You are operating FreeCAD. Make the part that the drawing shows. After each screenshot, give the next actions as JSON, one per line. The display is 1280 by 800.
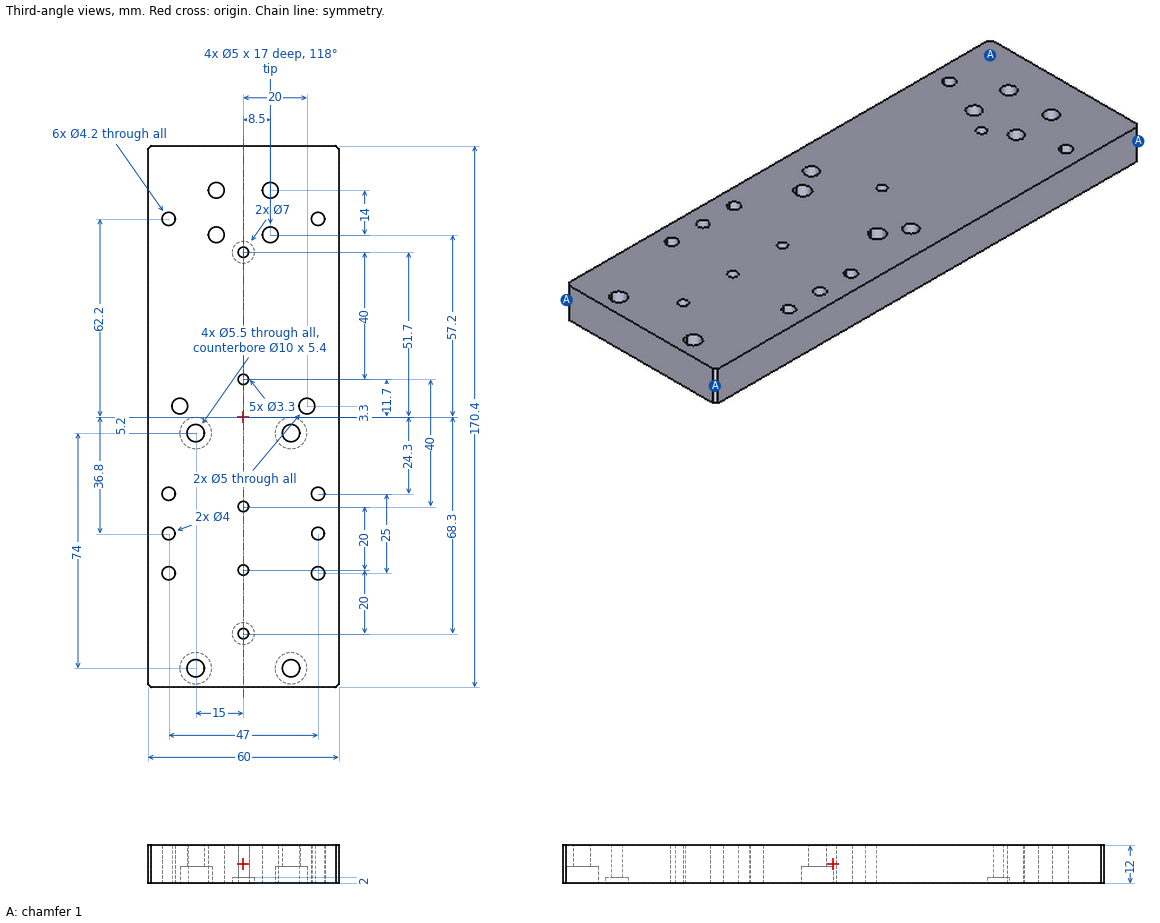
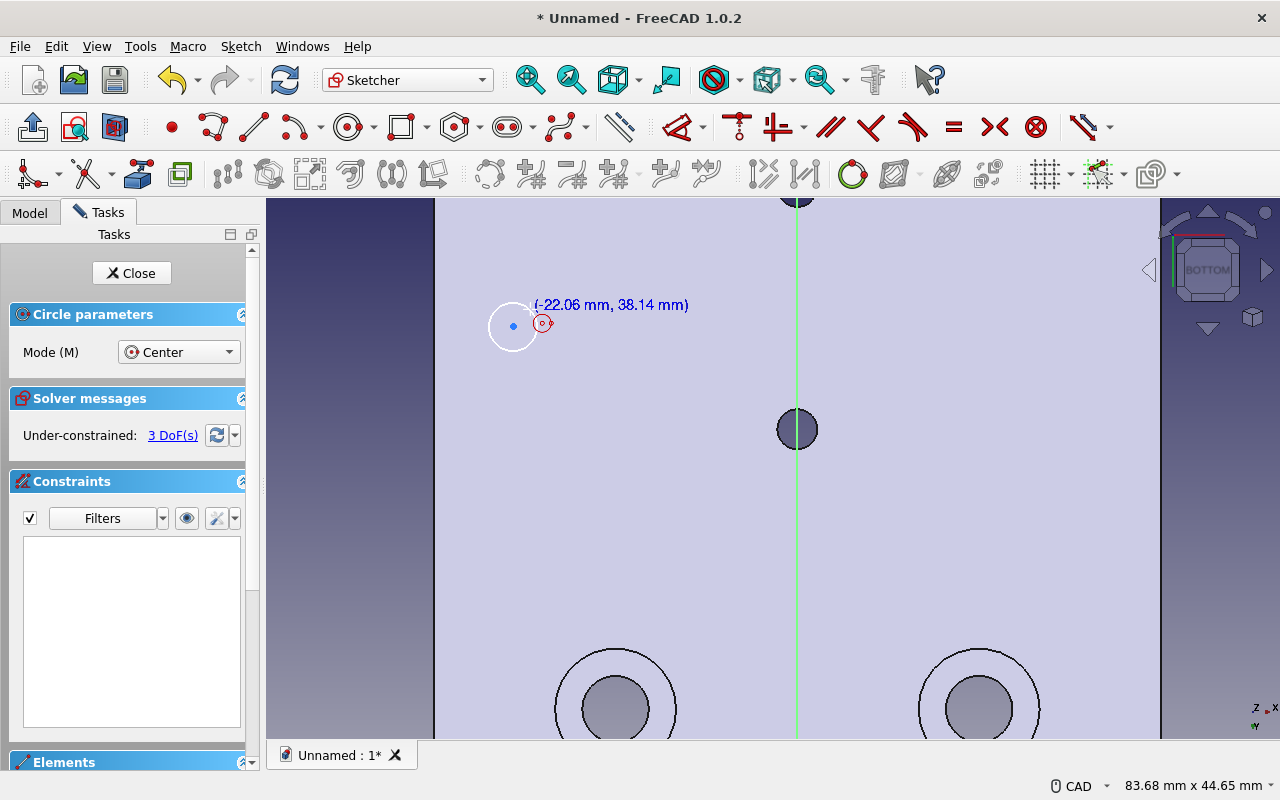
{"action": "left_click", "coordinate": [1082, 326]}
{"action": "left_click", "coordinate": [1099, 309]}
{"action": "key", "text": "Escape"}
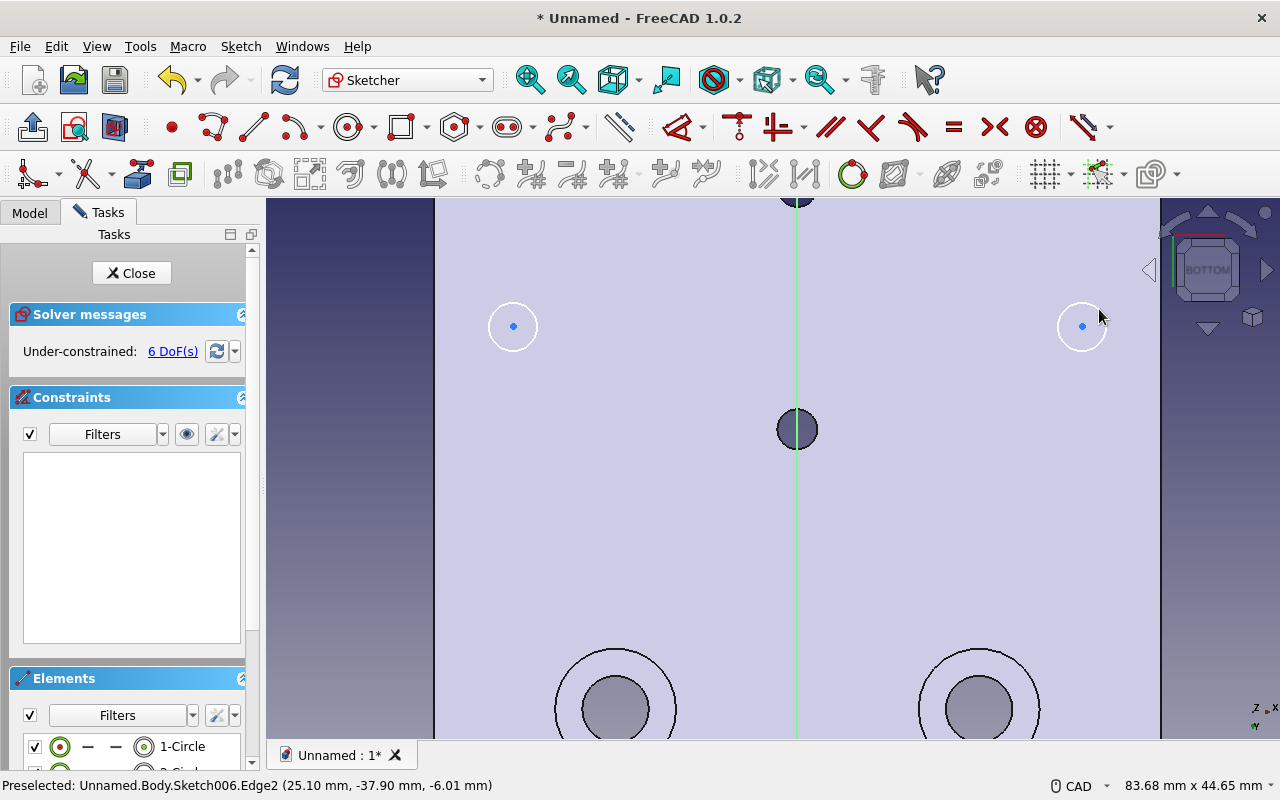
{"action": "left_click", "coordinate": [530, 310]}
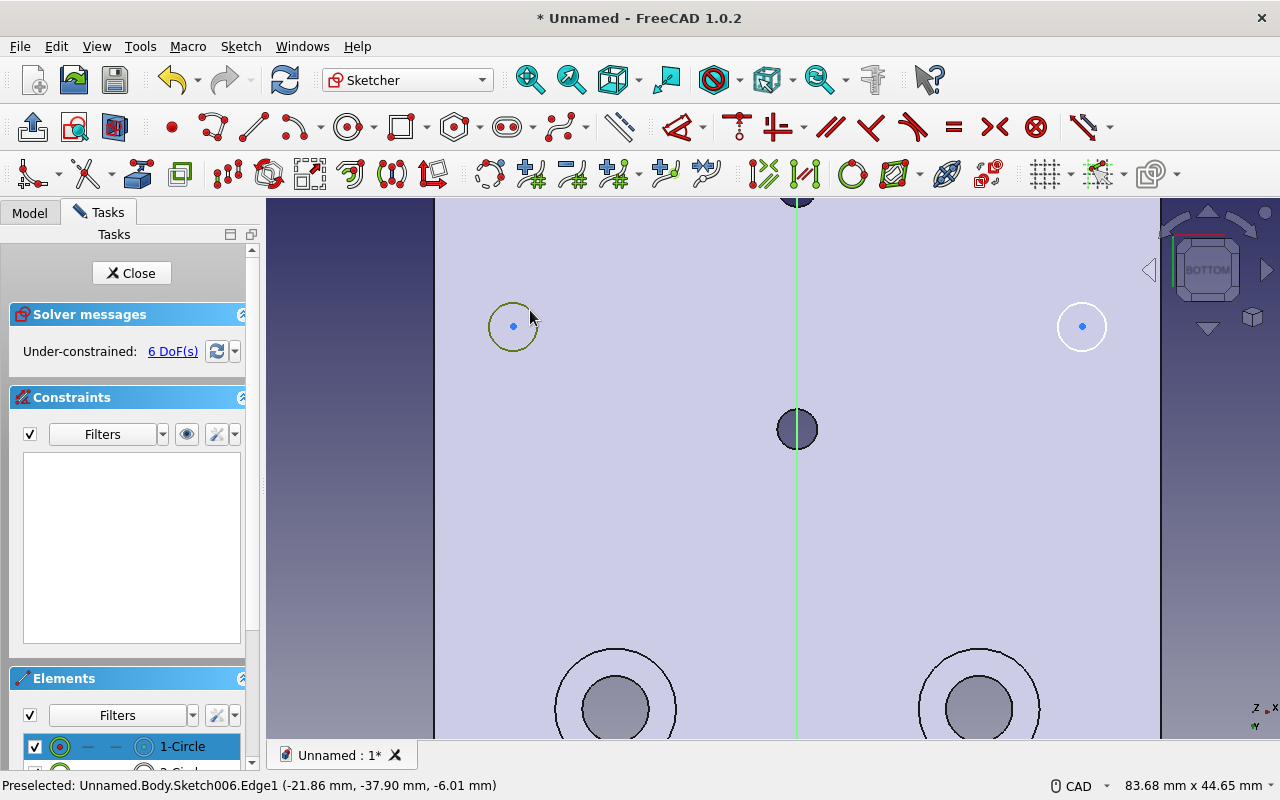
{"action": "left_click", "coordinate": [1099, 310]}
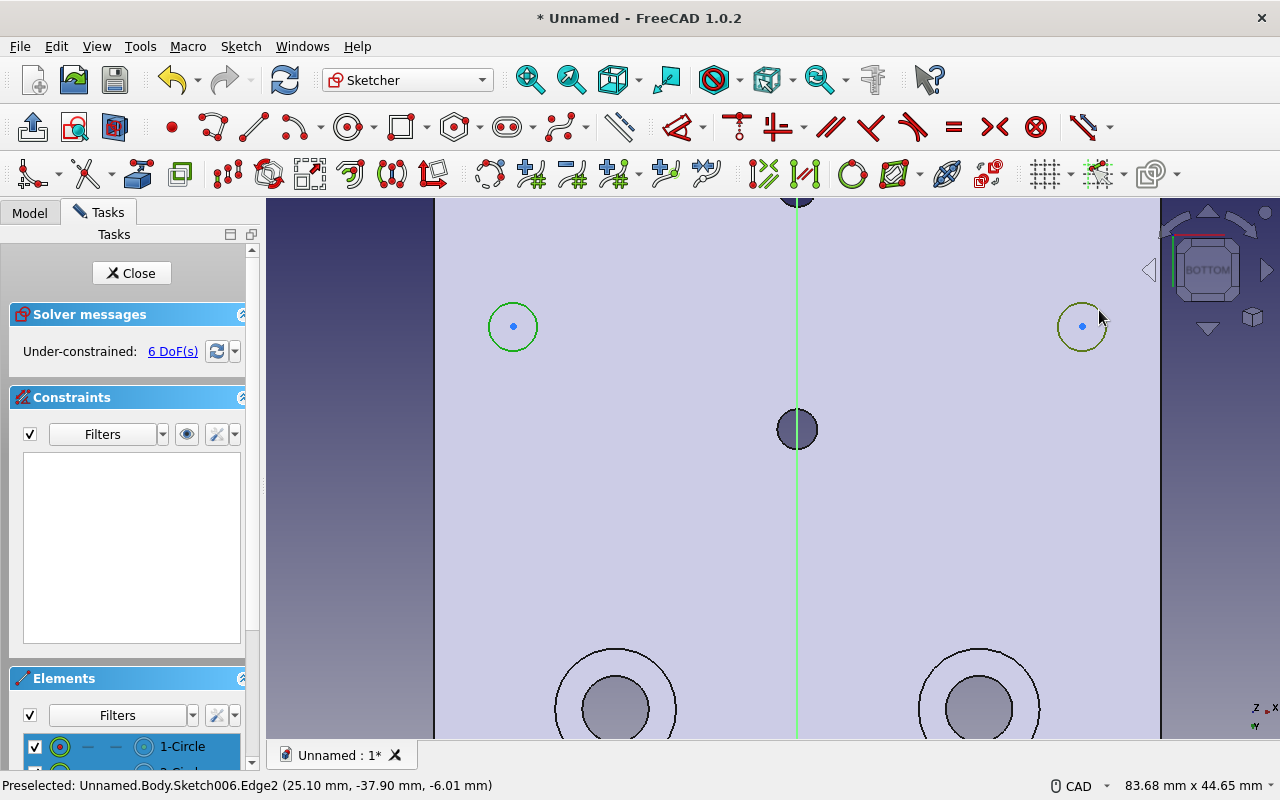
{"action": "left_click", "coordinate": [954, 128]}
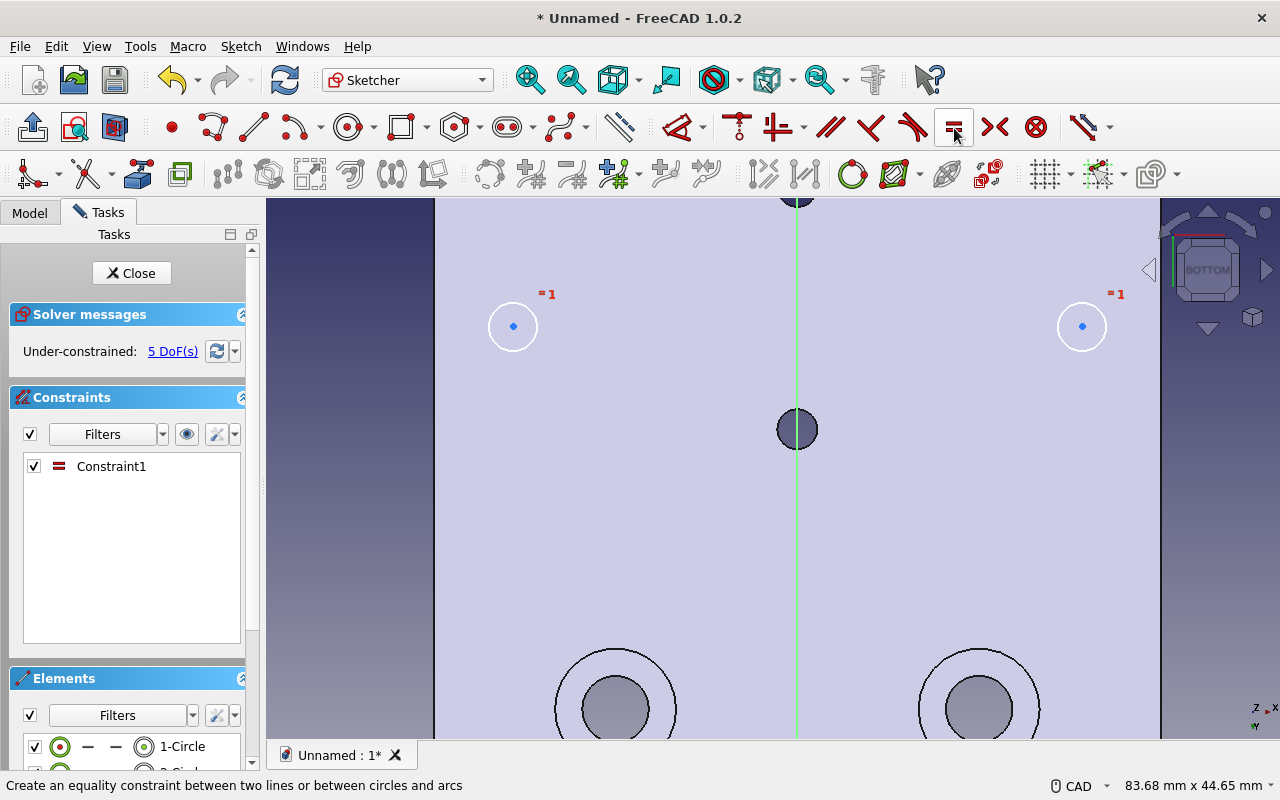
{"action": "left_click", "coordinate": [513, 327]}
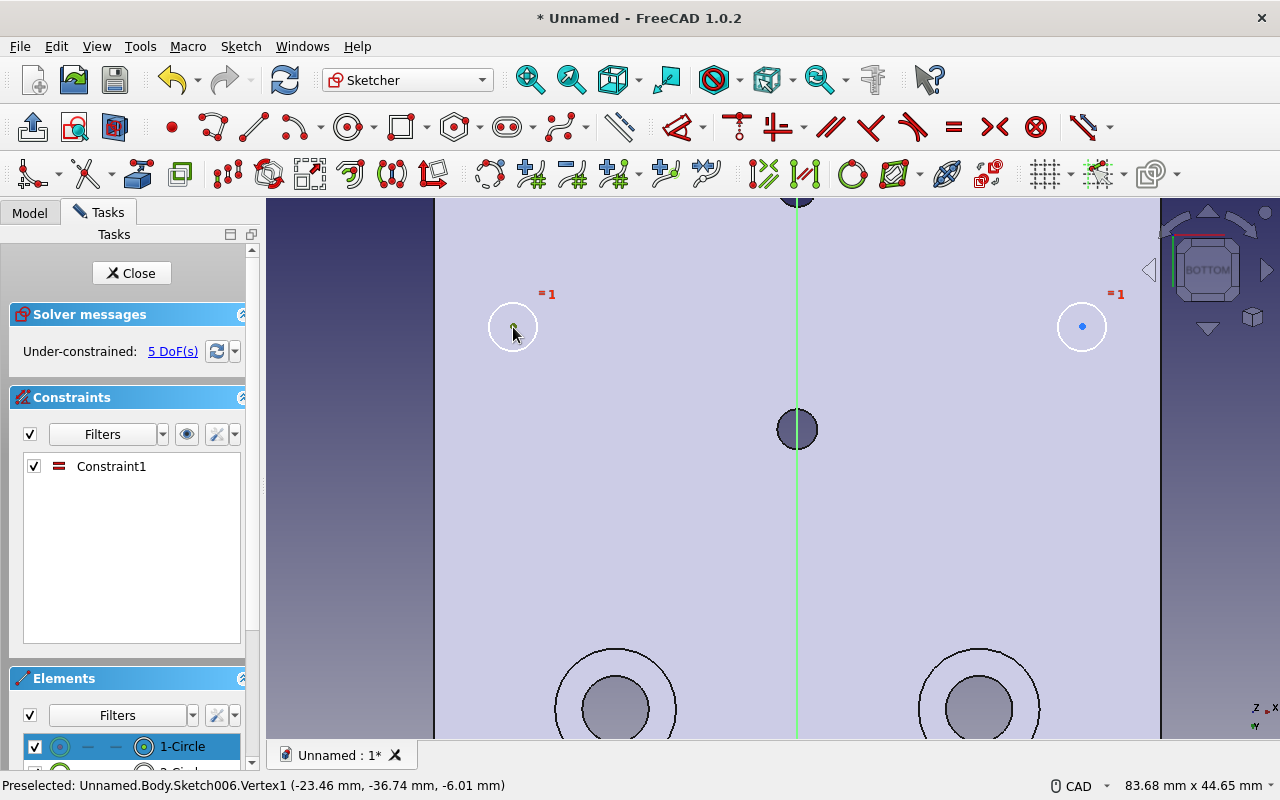
{"action": "left_click", "coordinate": [1082, 327]}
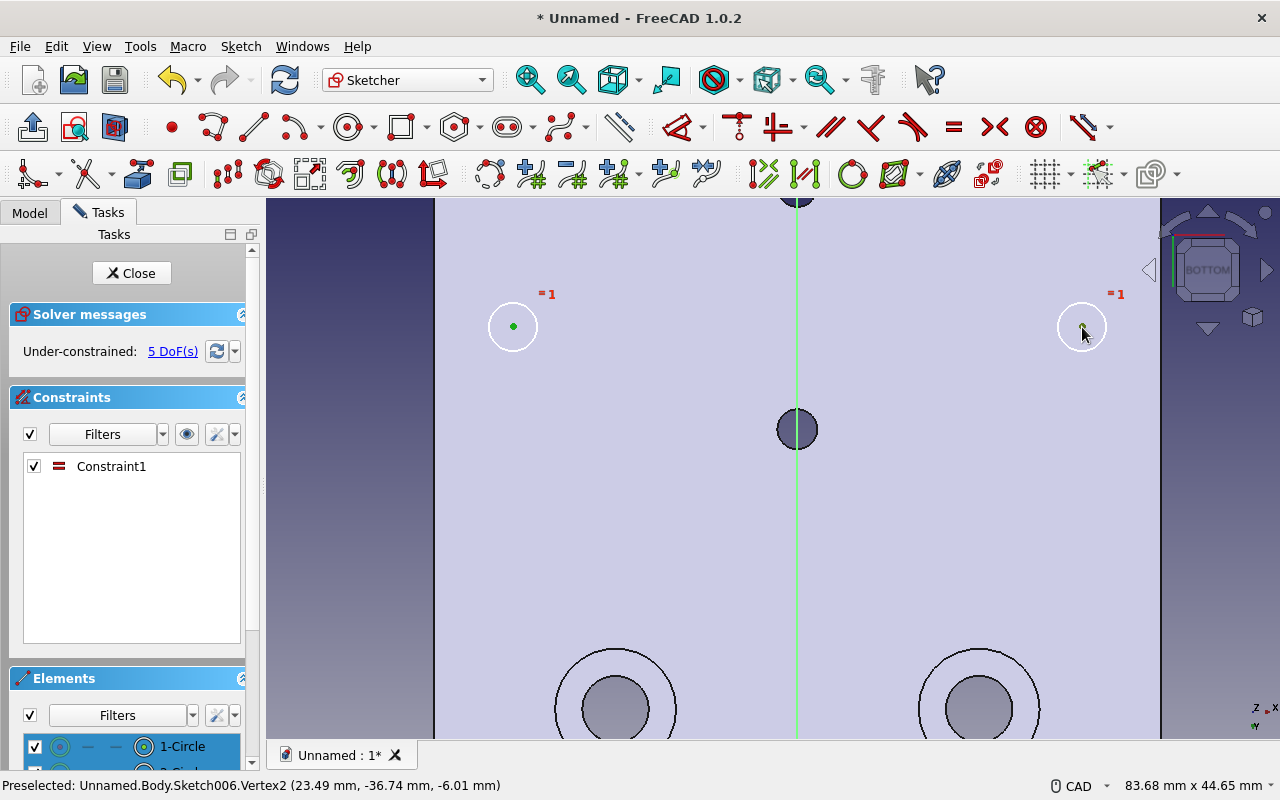
{"action": "left_click", "coordinate": [797, 676]}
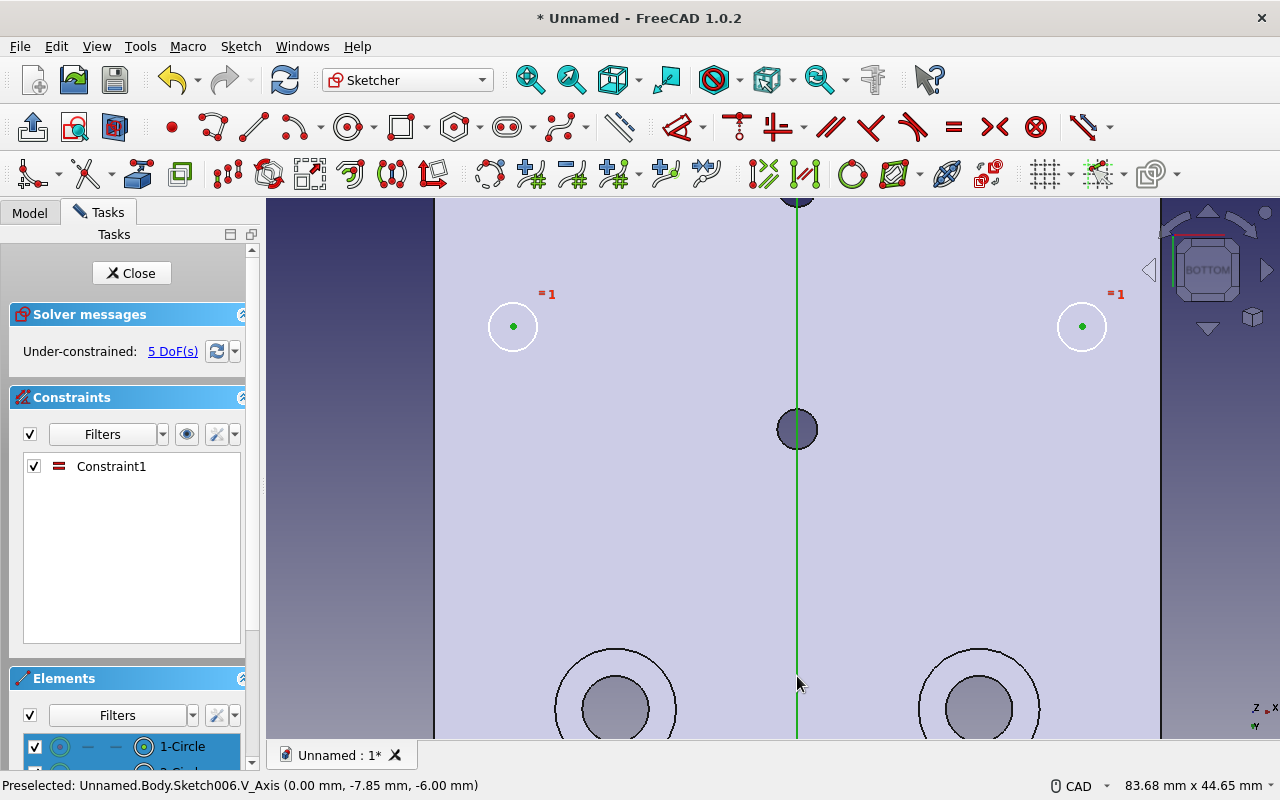
{"action": "left_click", "coordinate": [995, 128]}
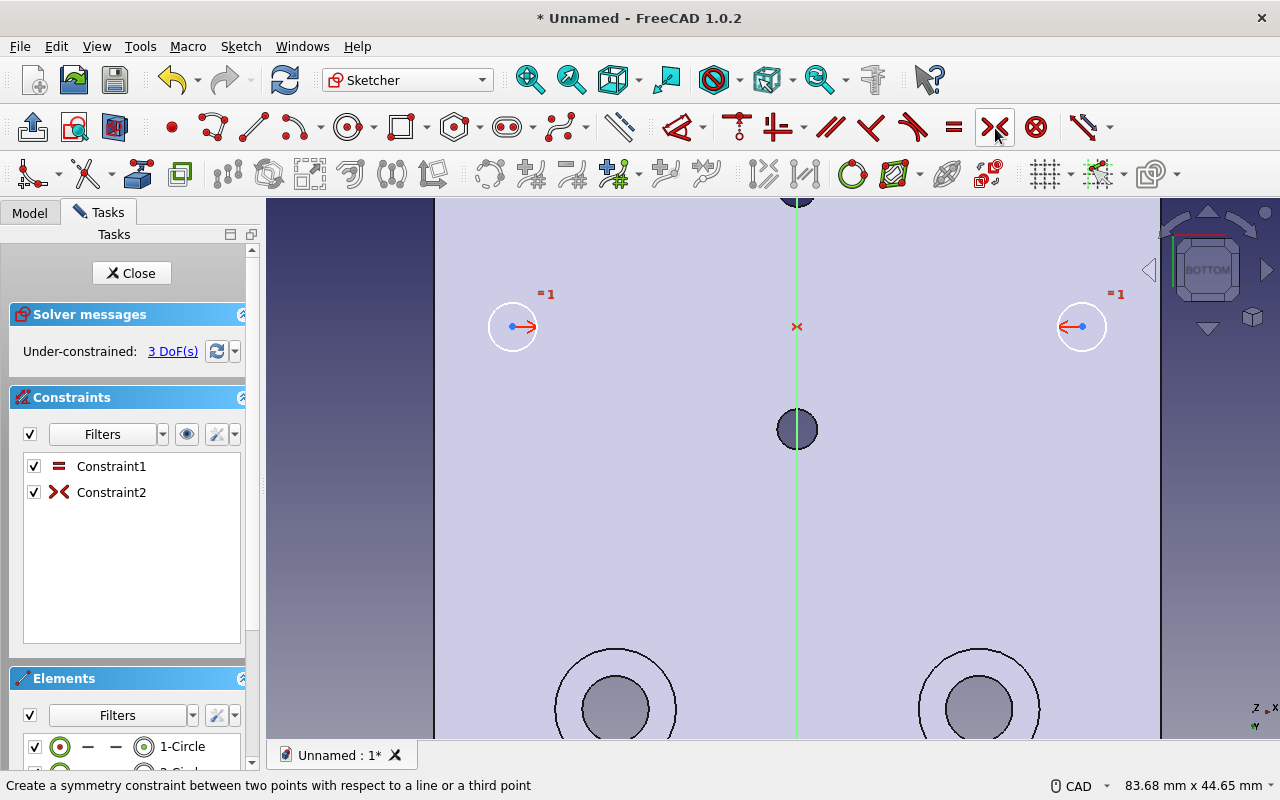
{"action": "left_click", "coordinate": [676, 128]}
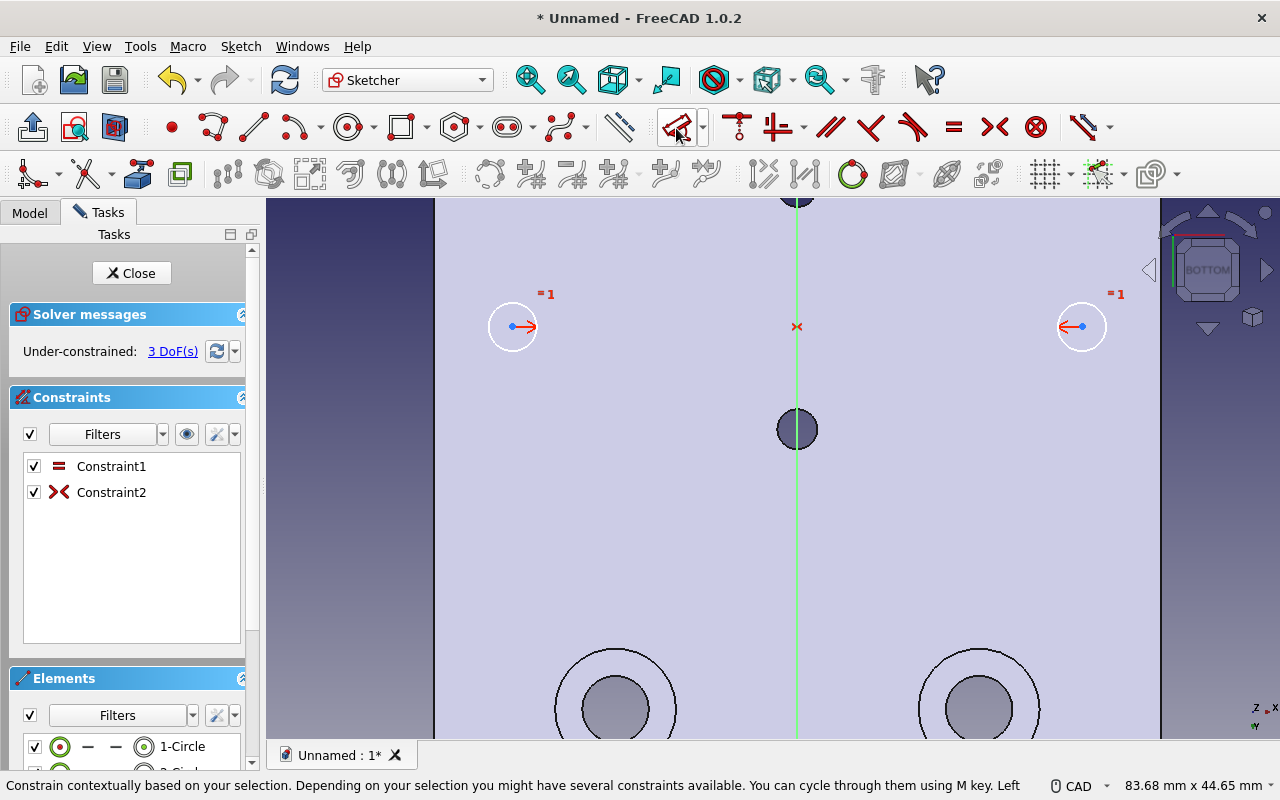
{"action": "left_click", "coordinate": [530, 310]}
{"action": "left_click", "coordinate": [553, 288]}